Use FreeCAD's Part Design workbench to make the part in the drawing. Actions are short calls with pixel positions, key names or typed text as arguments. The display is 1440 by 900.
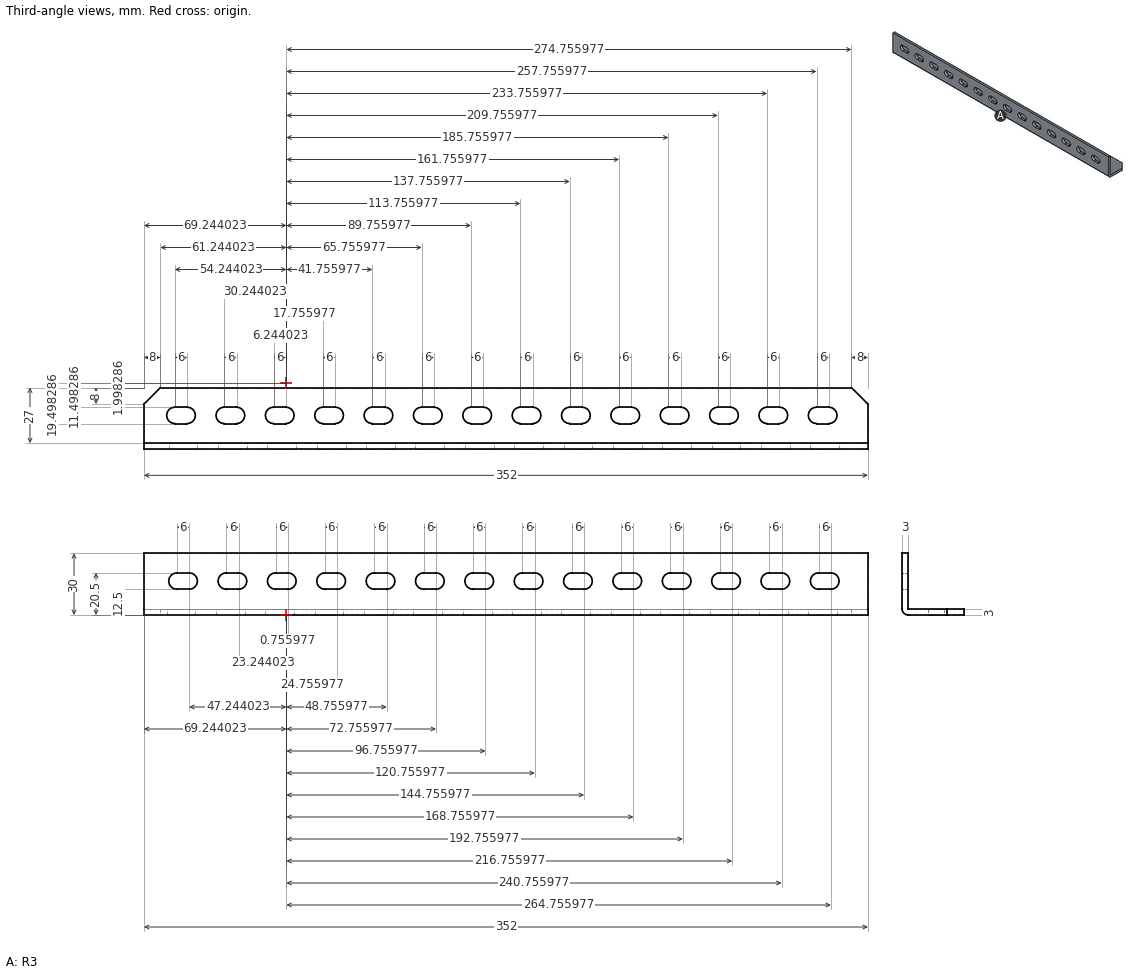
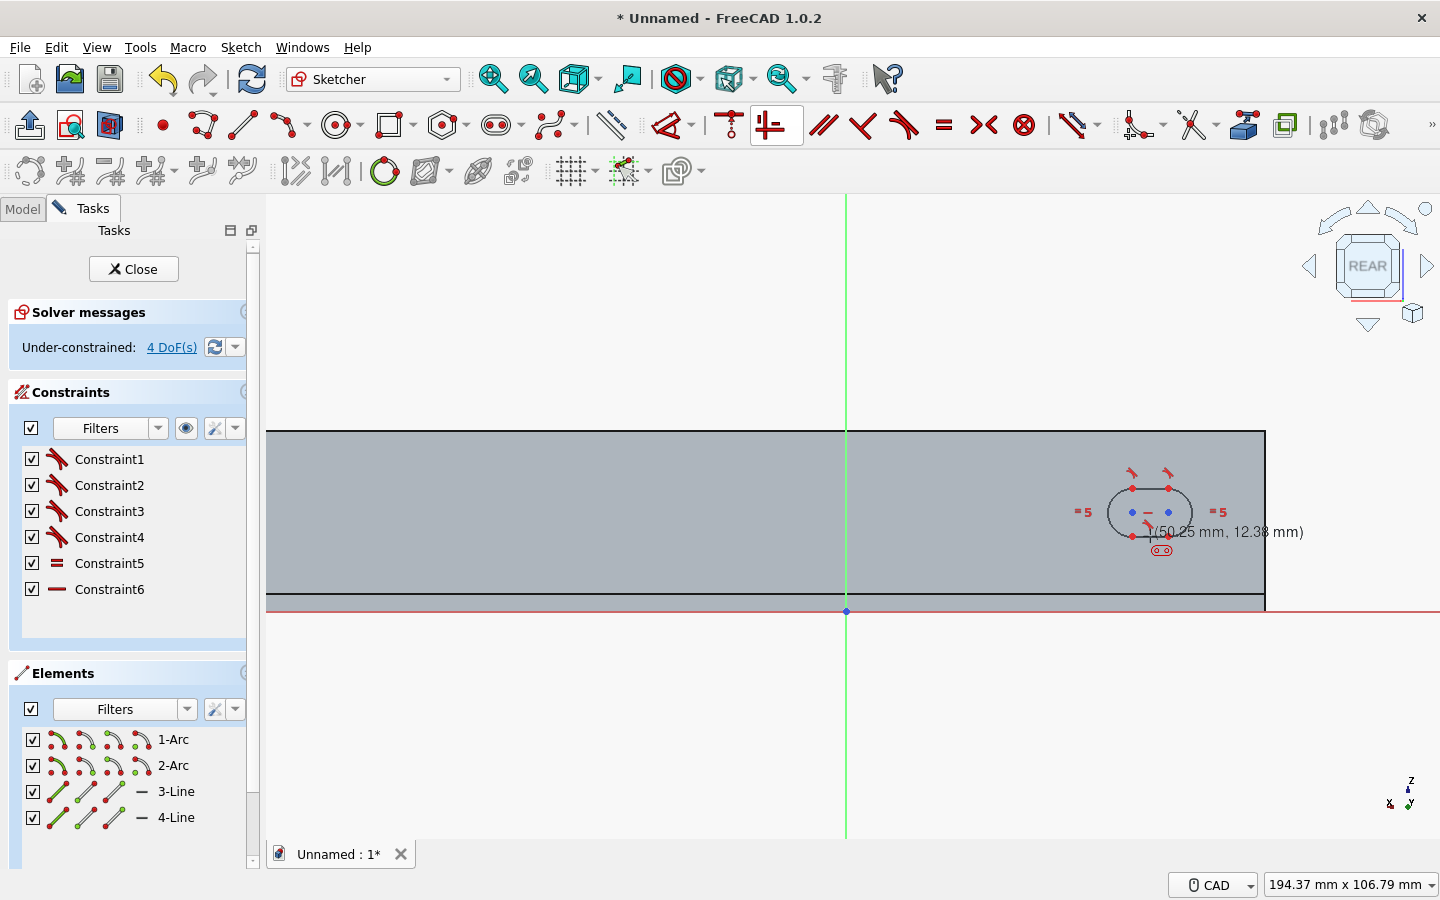
click(987, 512)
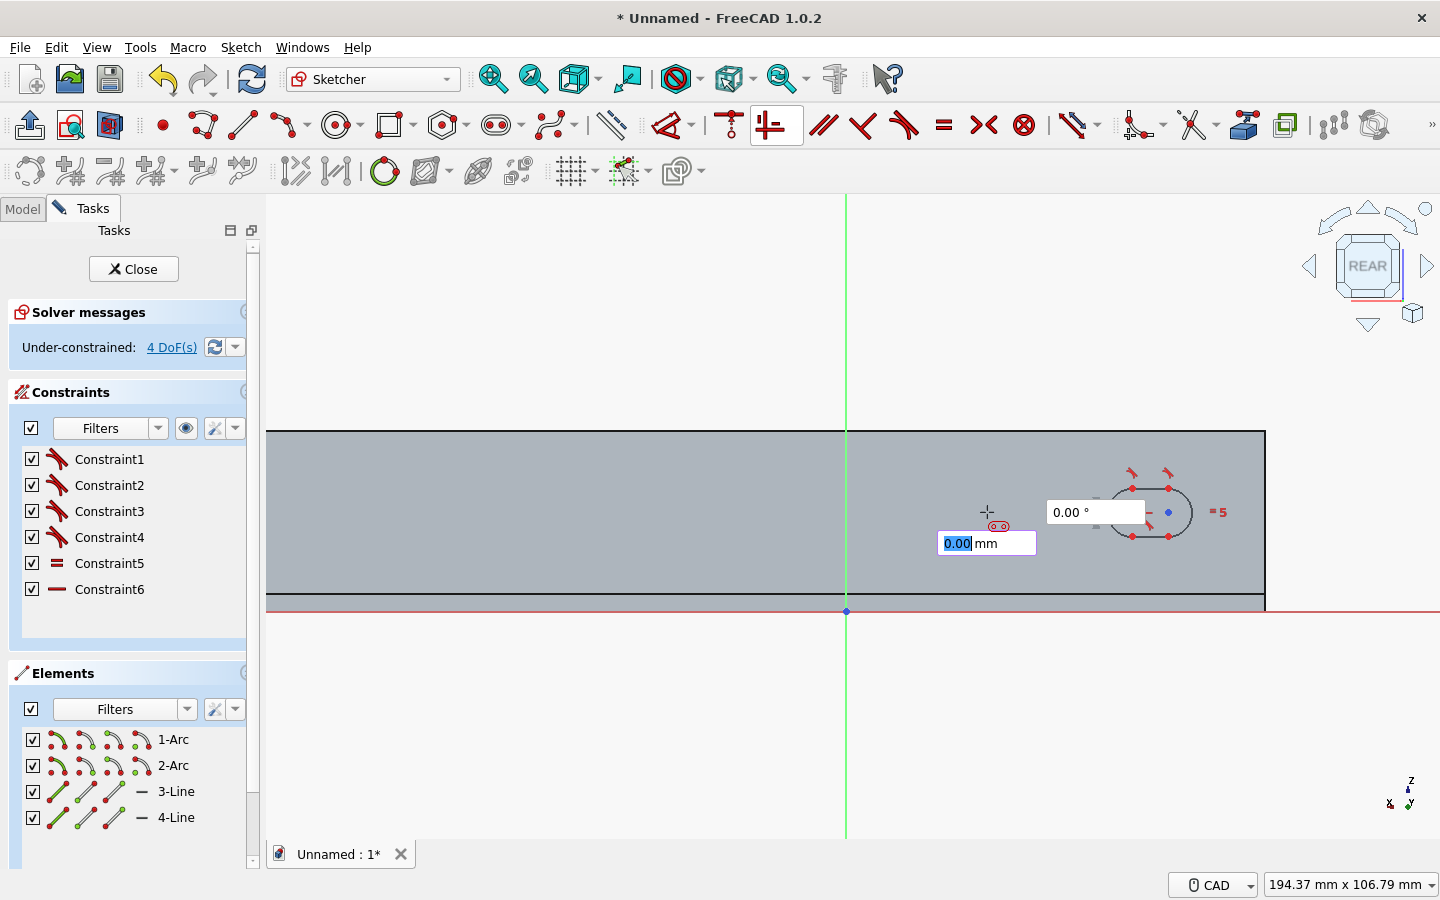
click(1023, 512)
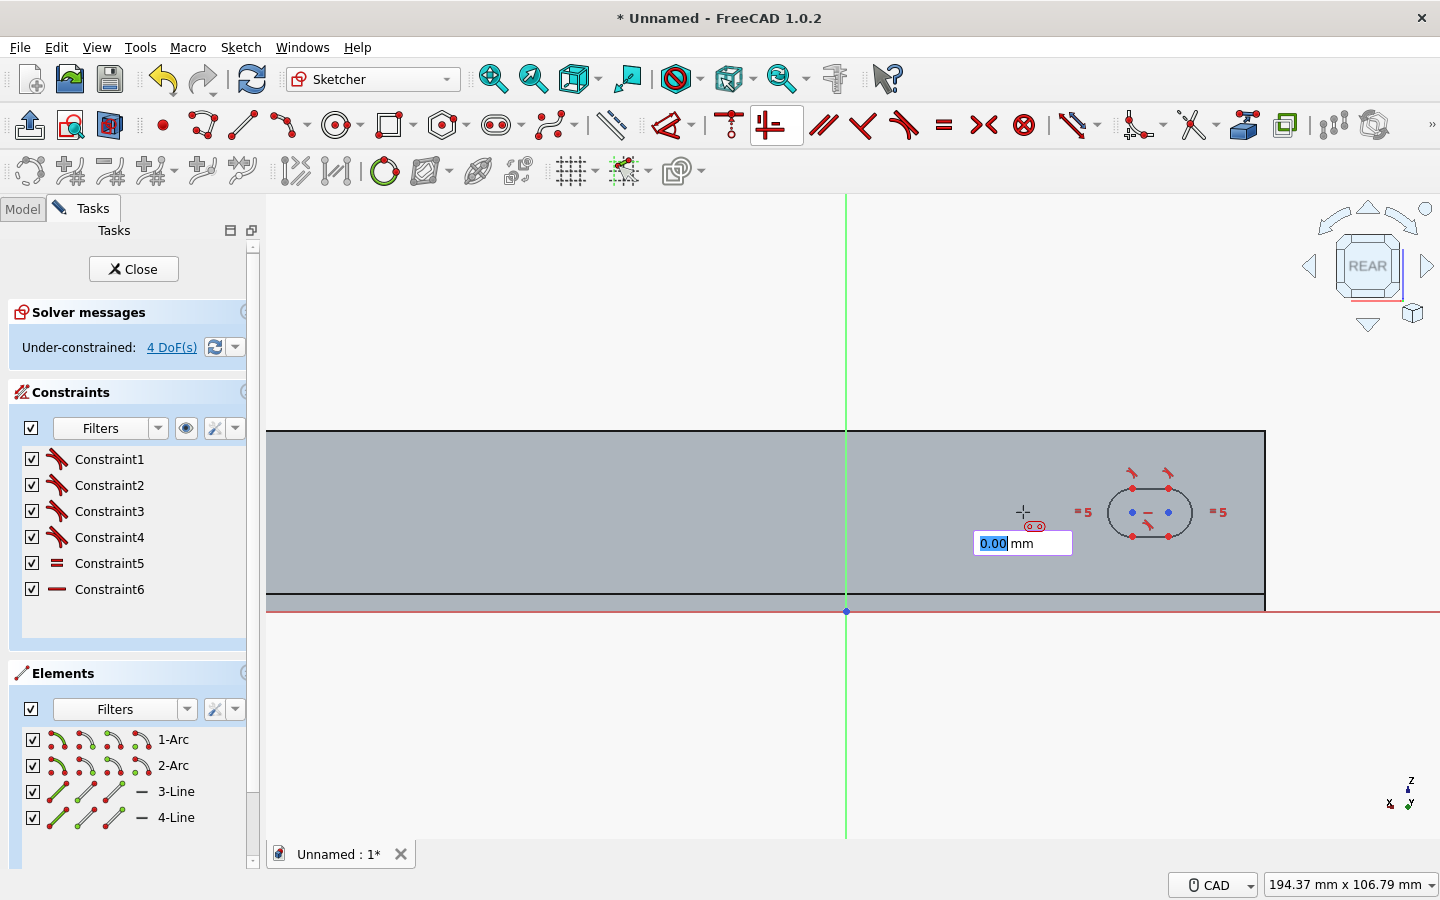
click(1005, 536)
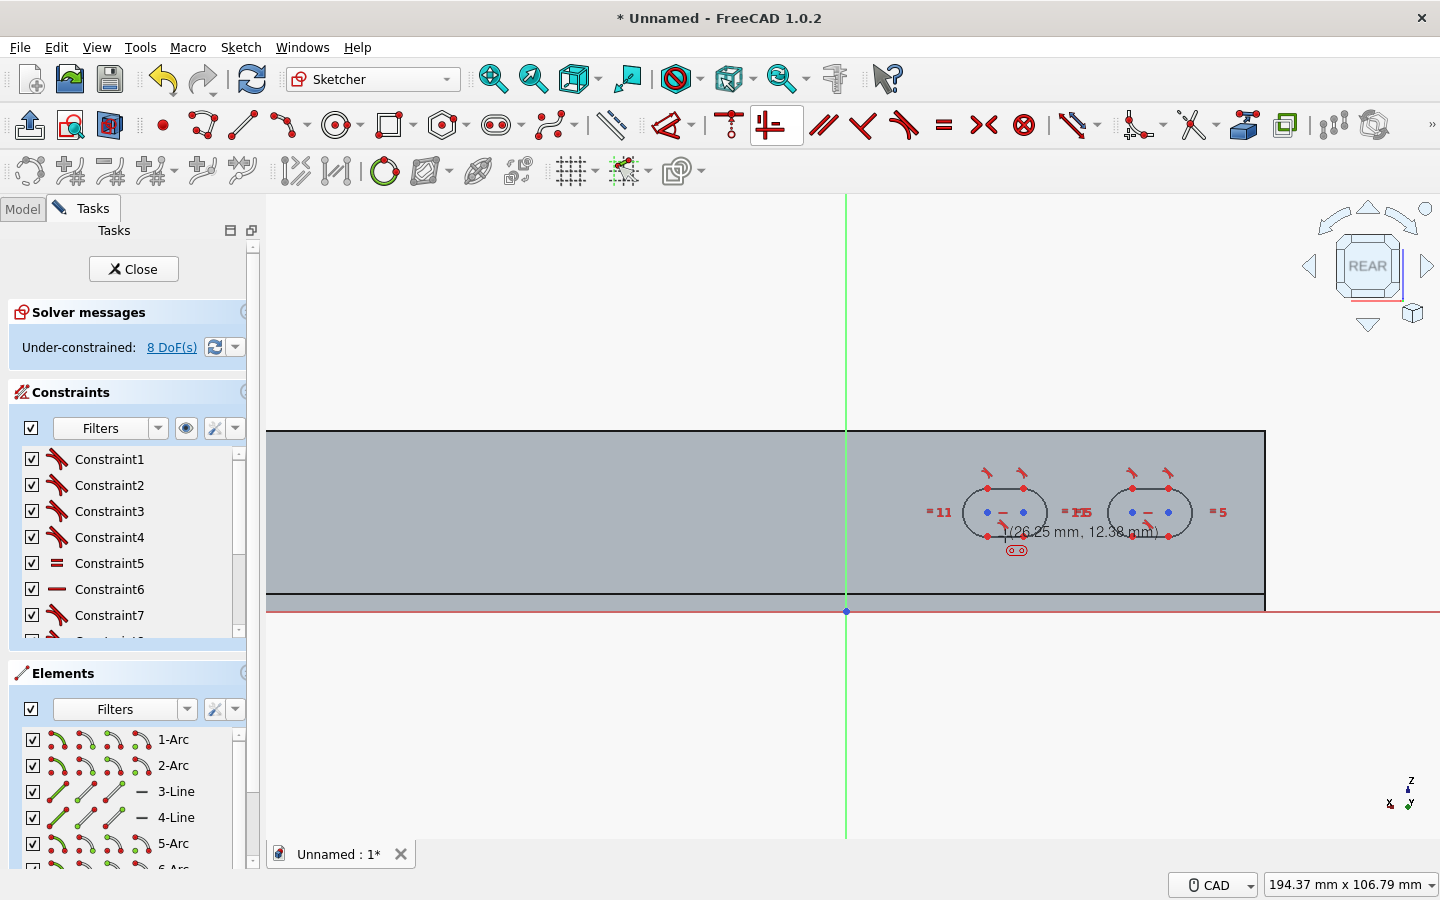
scroll(842, 512, up, 7)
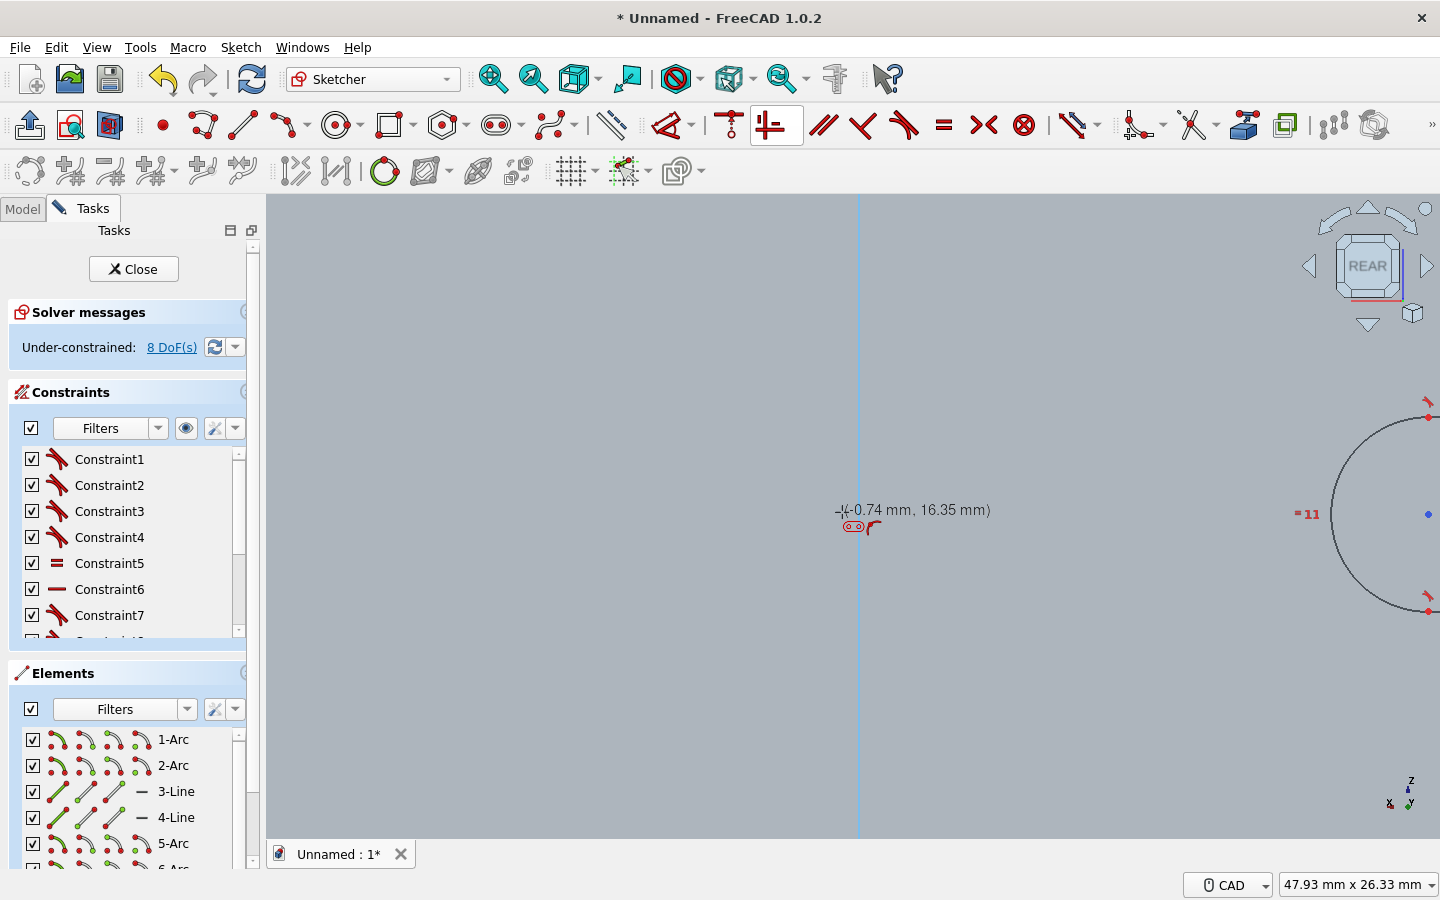
click(840, 511)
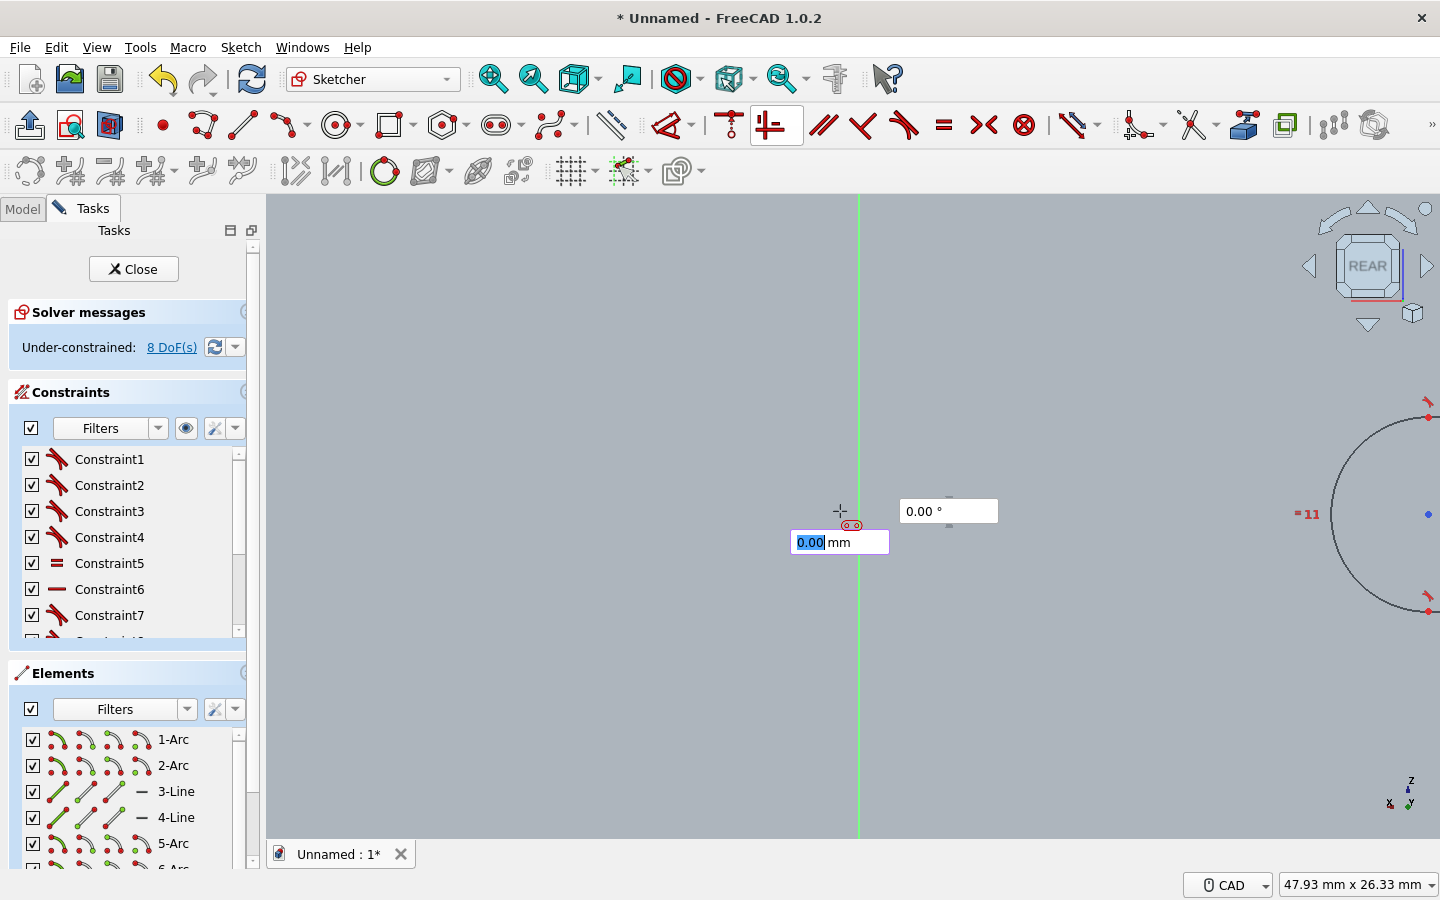
scroll(1036, 502, down, 12)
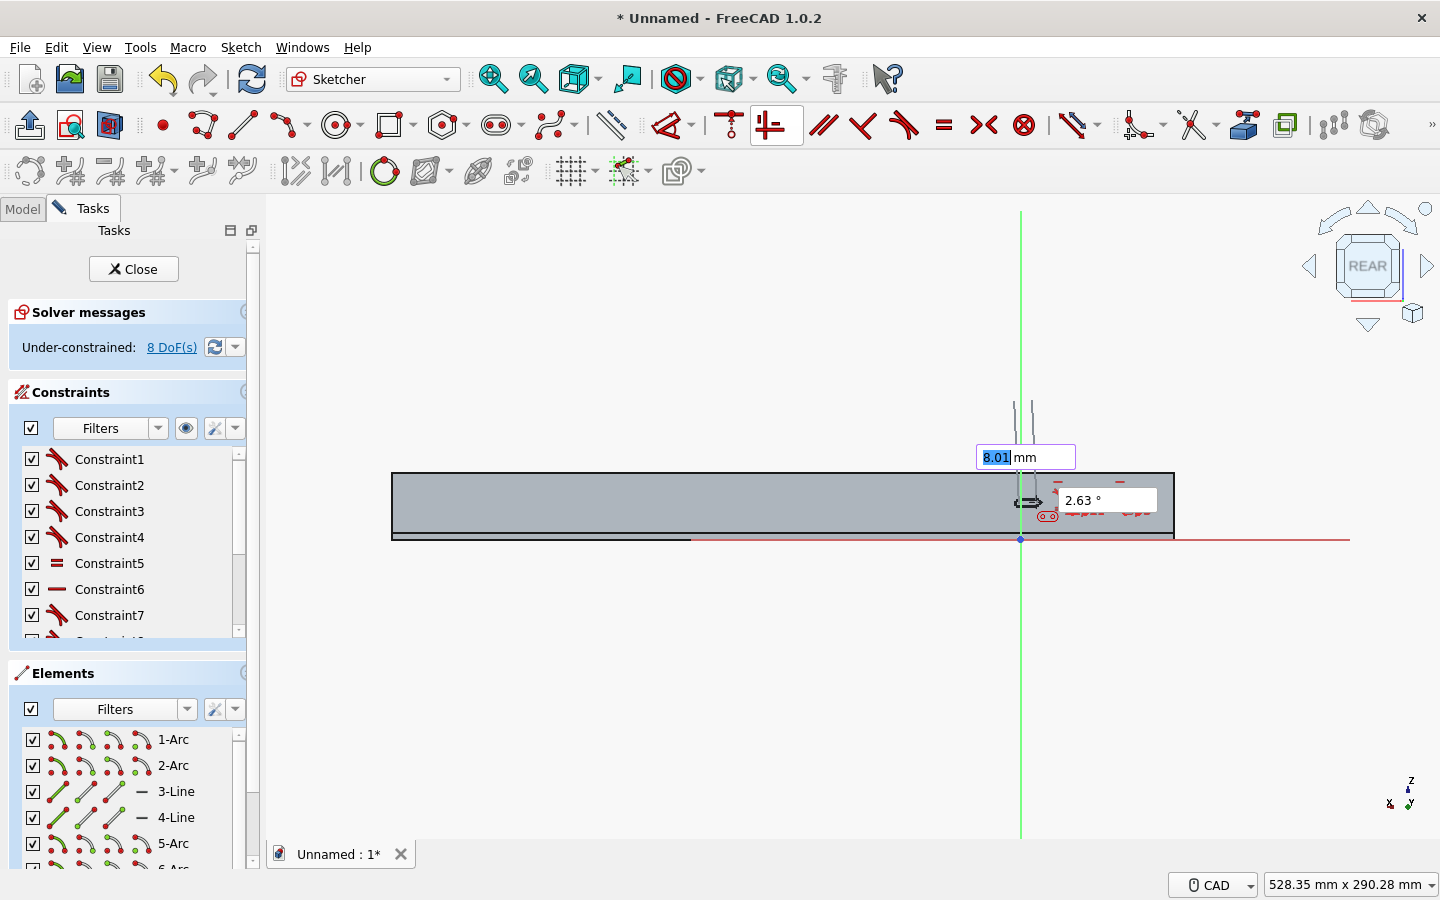
scroll(1032, 503, up, 2)